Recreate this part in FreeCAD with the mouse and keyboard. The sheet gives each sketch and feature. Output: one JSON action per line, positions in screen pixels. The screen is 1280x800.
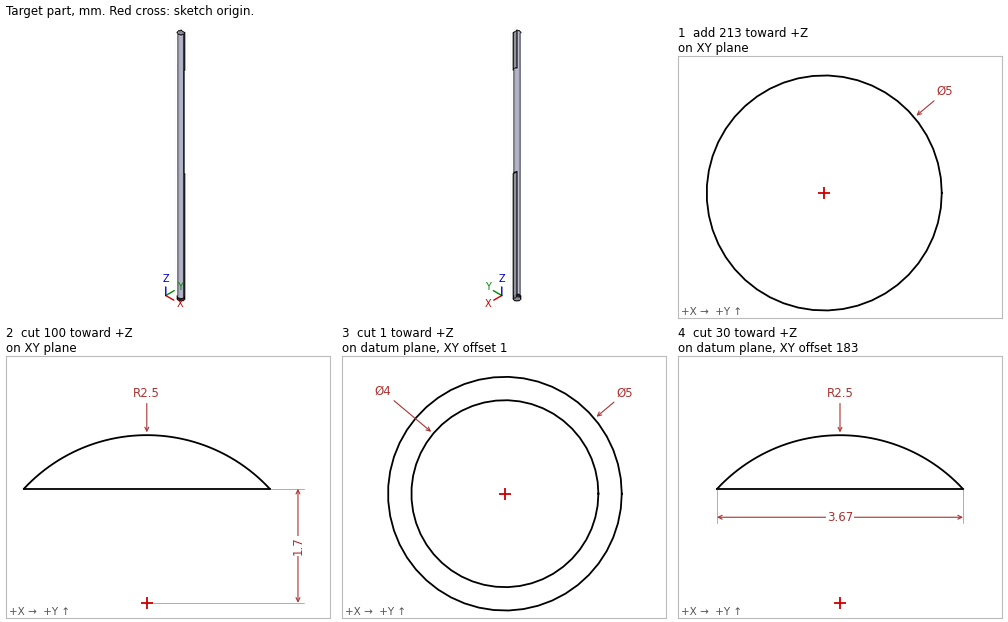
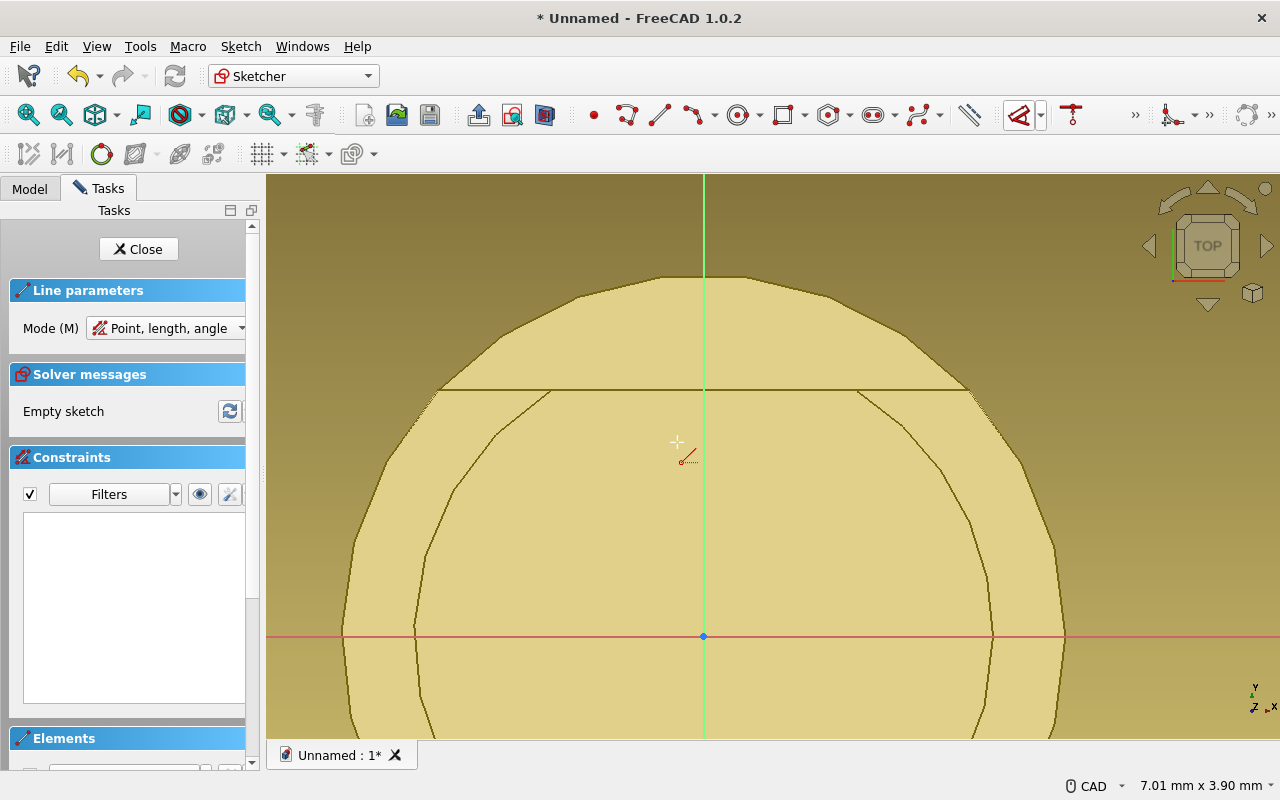
{"action": "left_click", "coordinate": [438, 391]}
{"action": "left_click", "coordinate": [969, 391]}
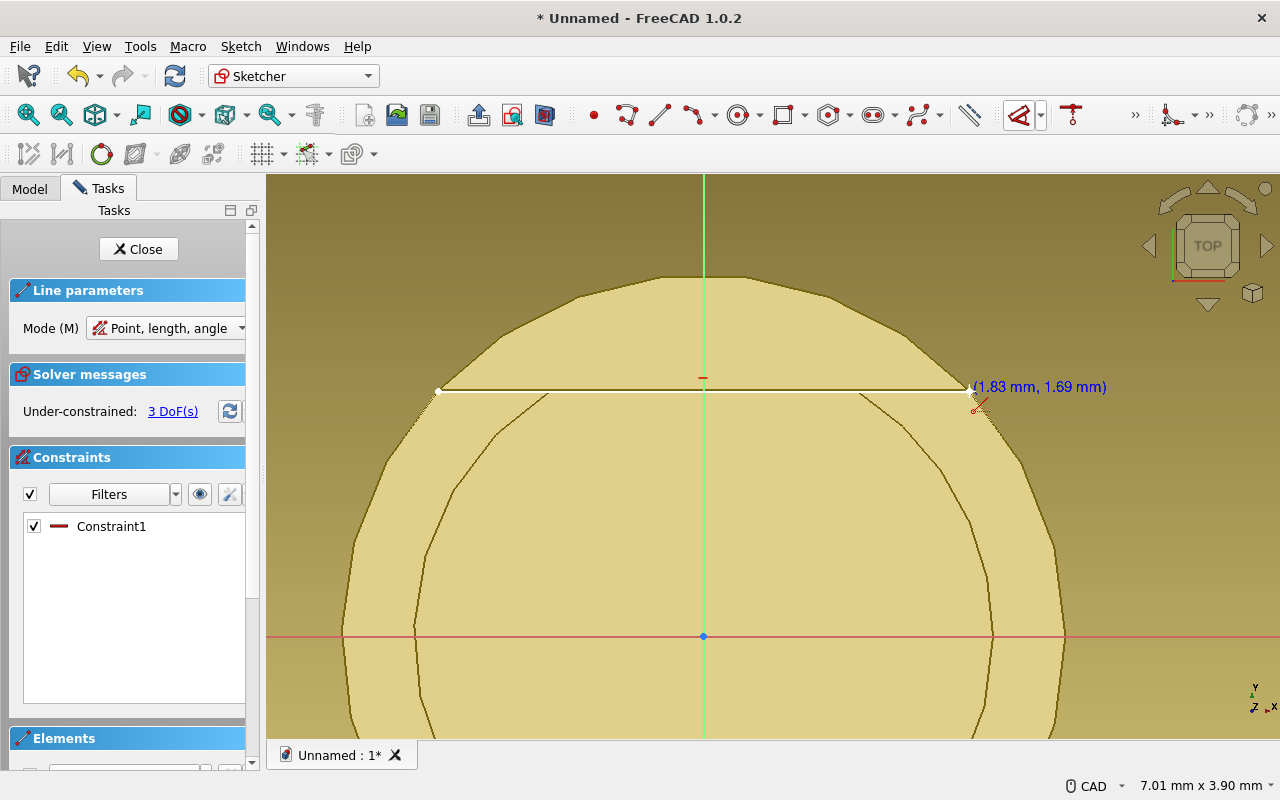
{"action": "key", "text": "g 3 a"}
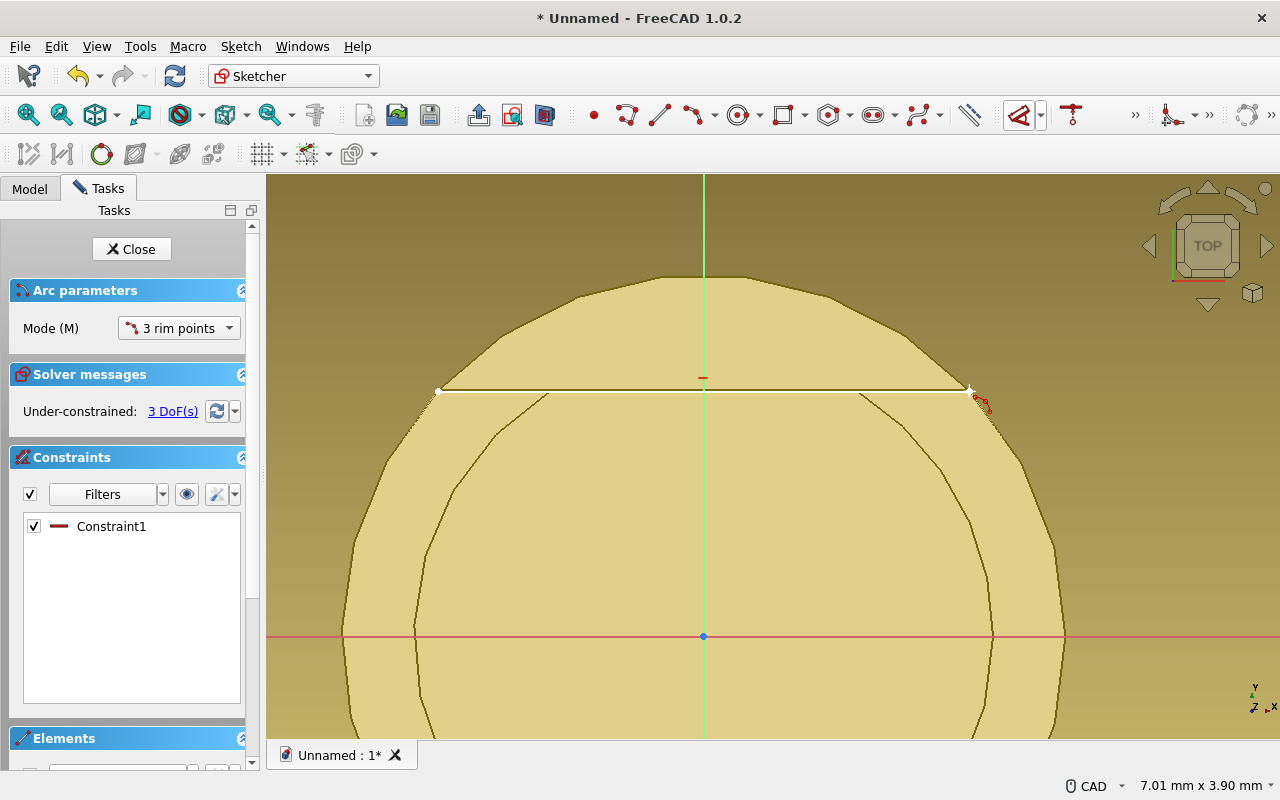
{"action": "left_click", "coordinate": [969, 392]}
{"action": "left_click", "coordinate": [438, 392]}
{"action": "left_click", "coordinate": [763, 280]}
{"action": "key", "text": "Escape"}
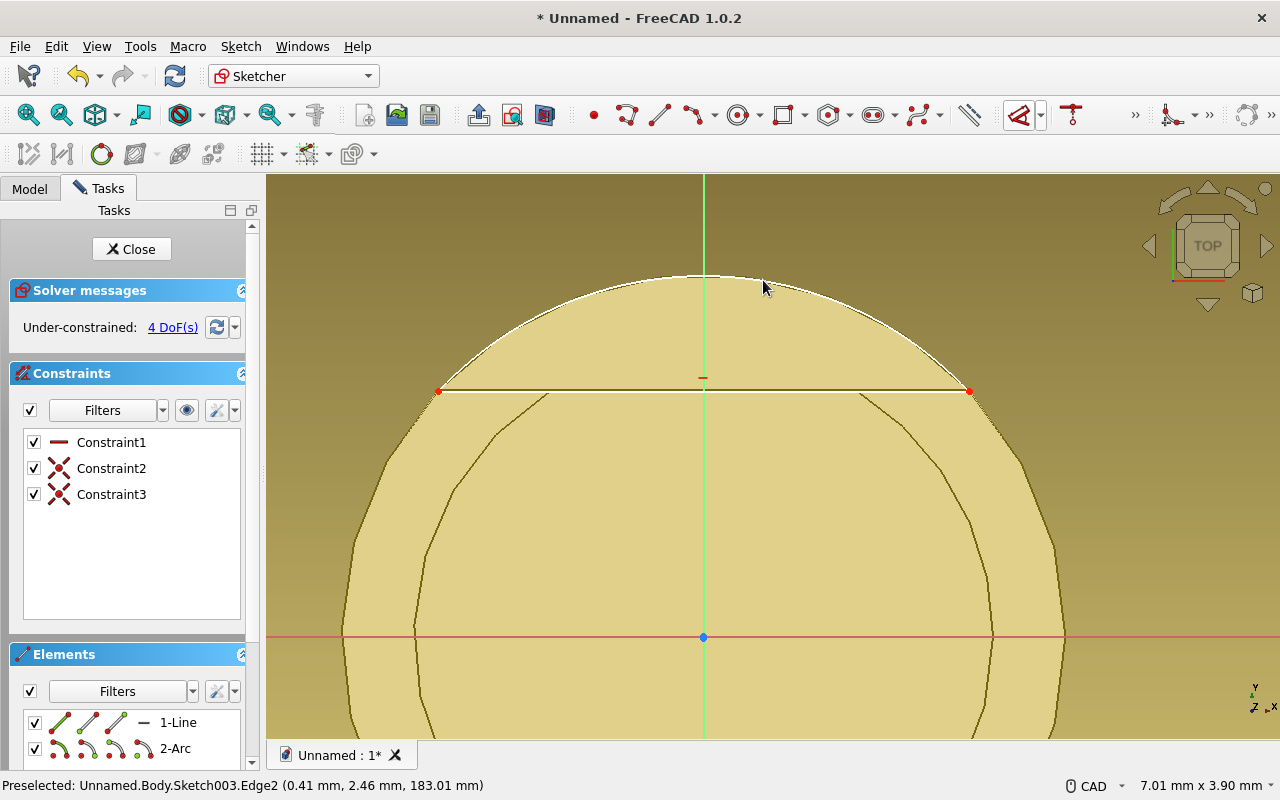
{"action": "left_click_drag", "start_coordinate": [694, 627], "coordinate": [714, 648]}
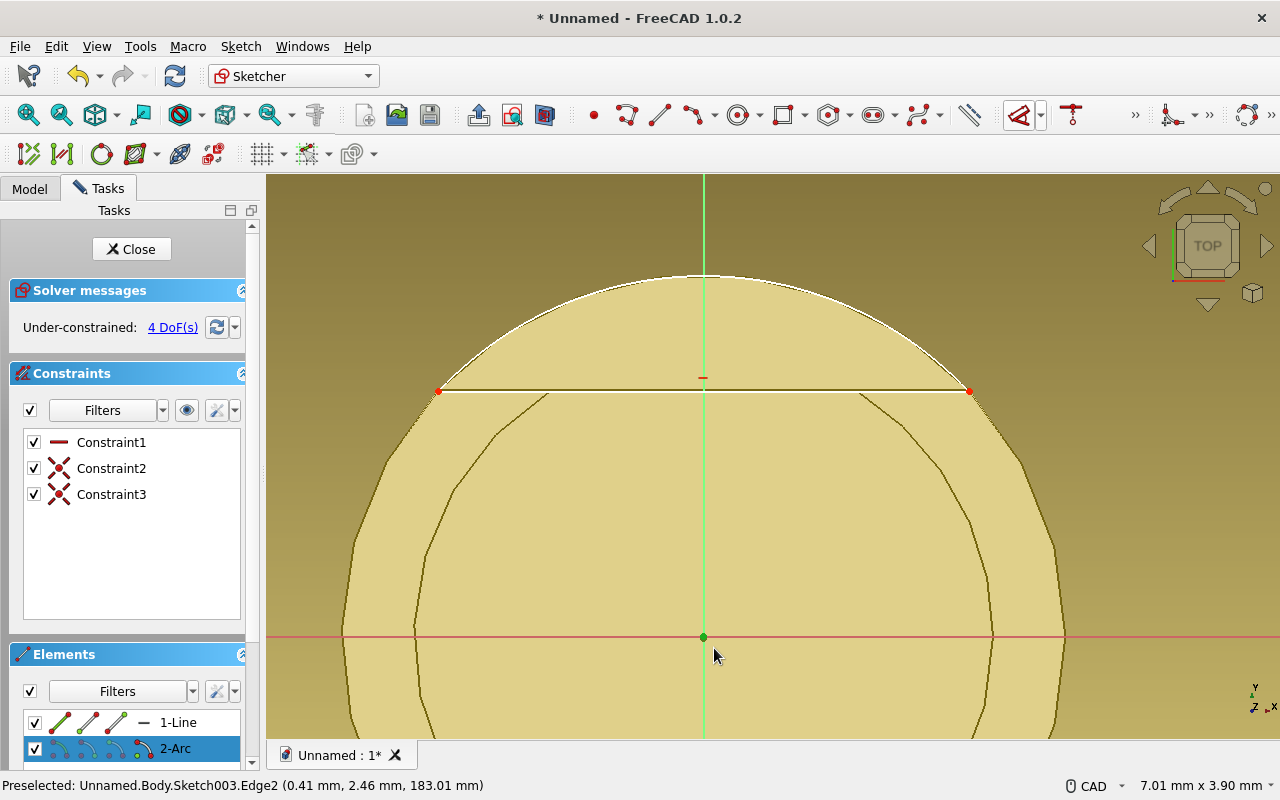
{"action": "key", "text": "c"}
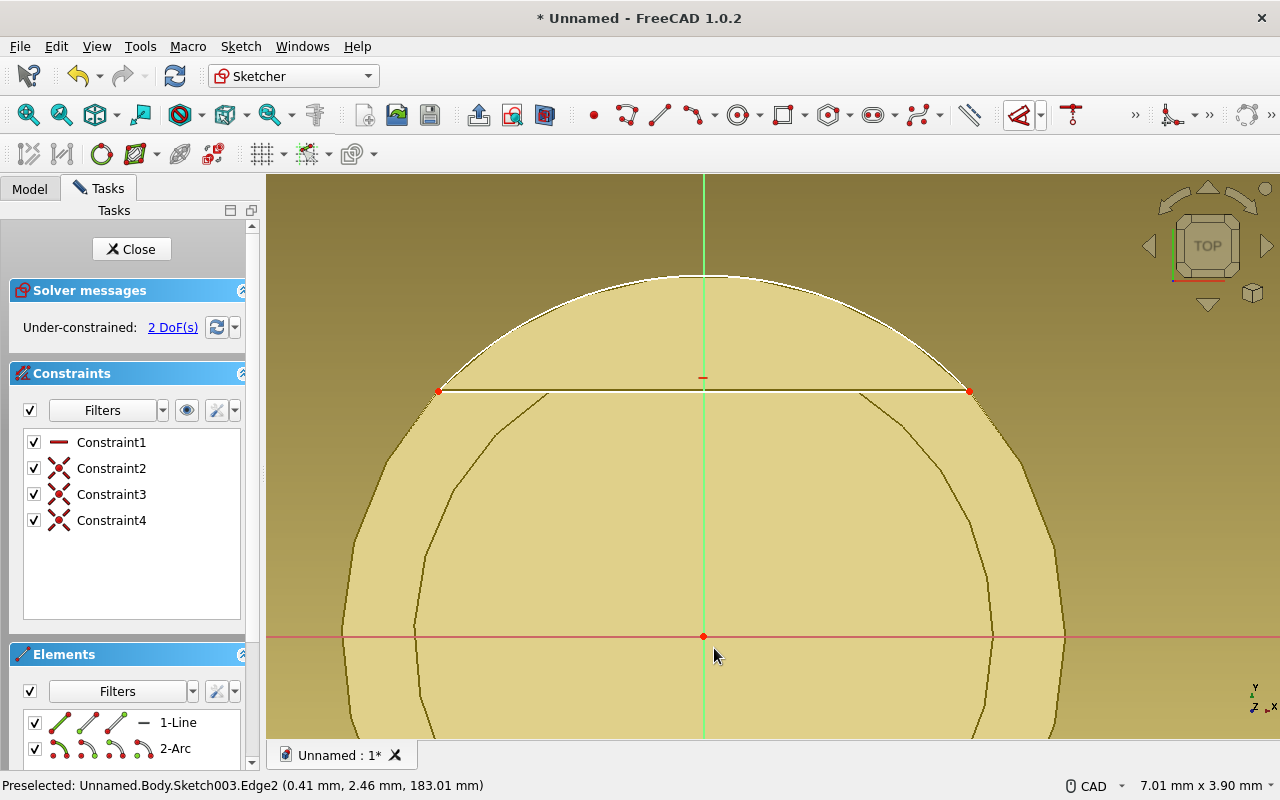
{"action": "left_click", "coordinate": [821, 295]}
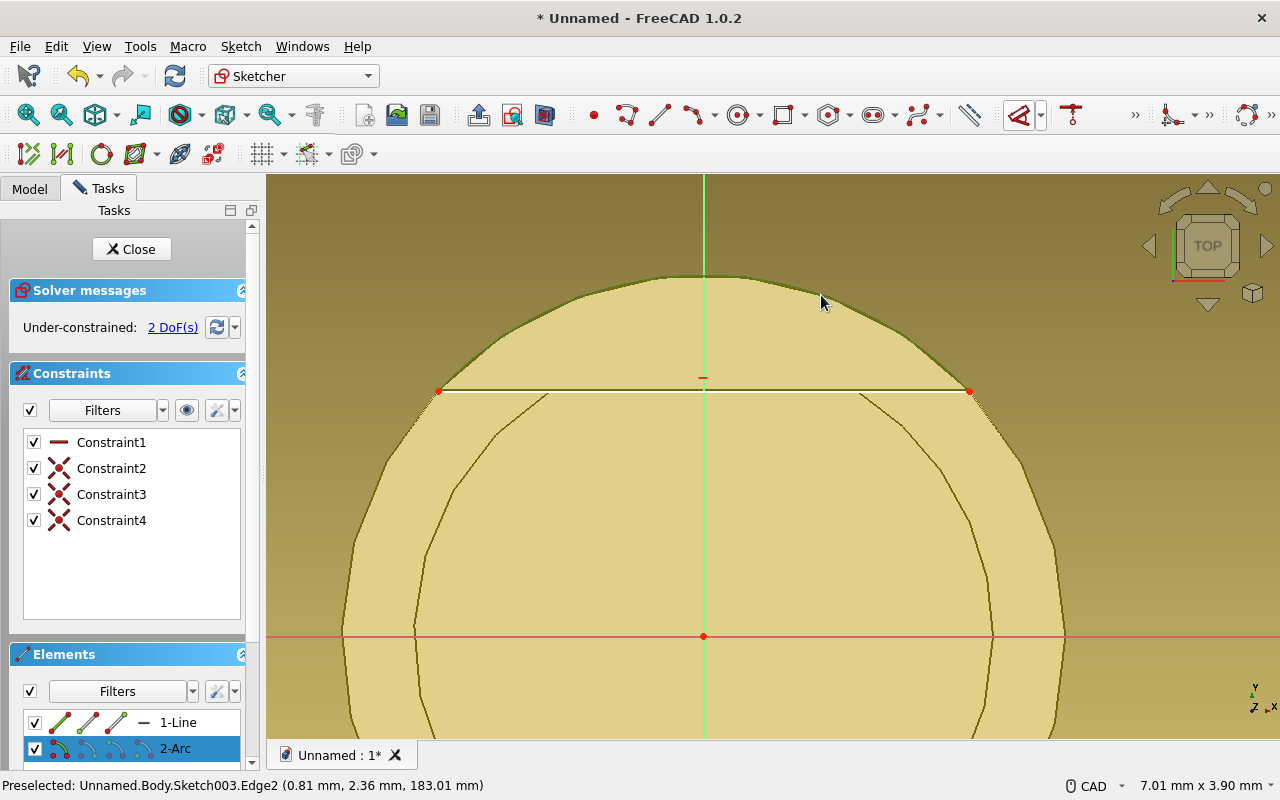
{"action": "key", "text": "k r"}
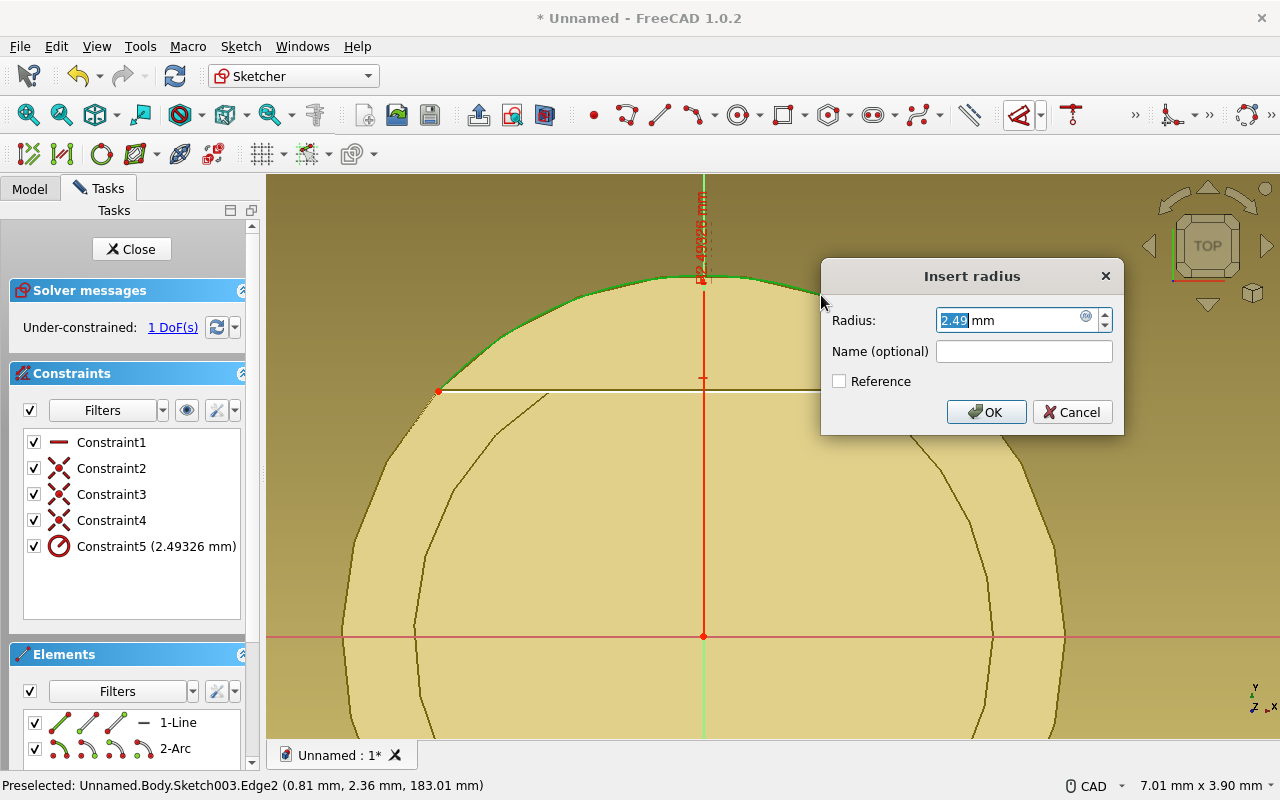
{"action": "type", "text": "2.5"}
{"action": "key", "text": "Return"}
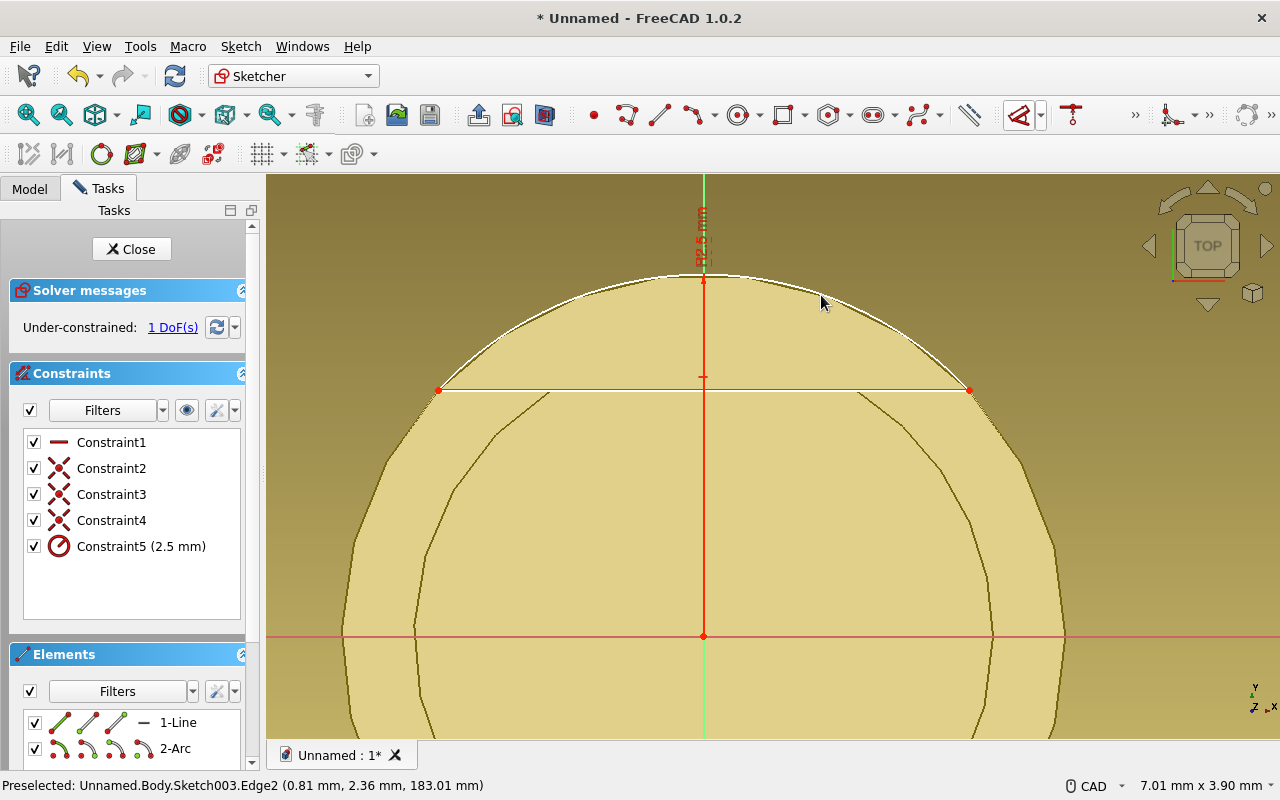
{"action": "left_click", "coordinate": [597, 391]}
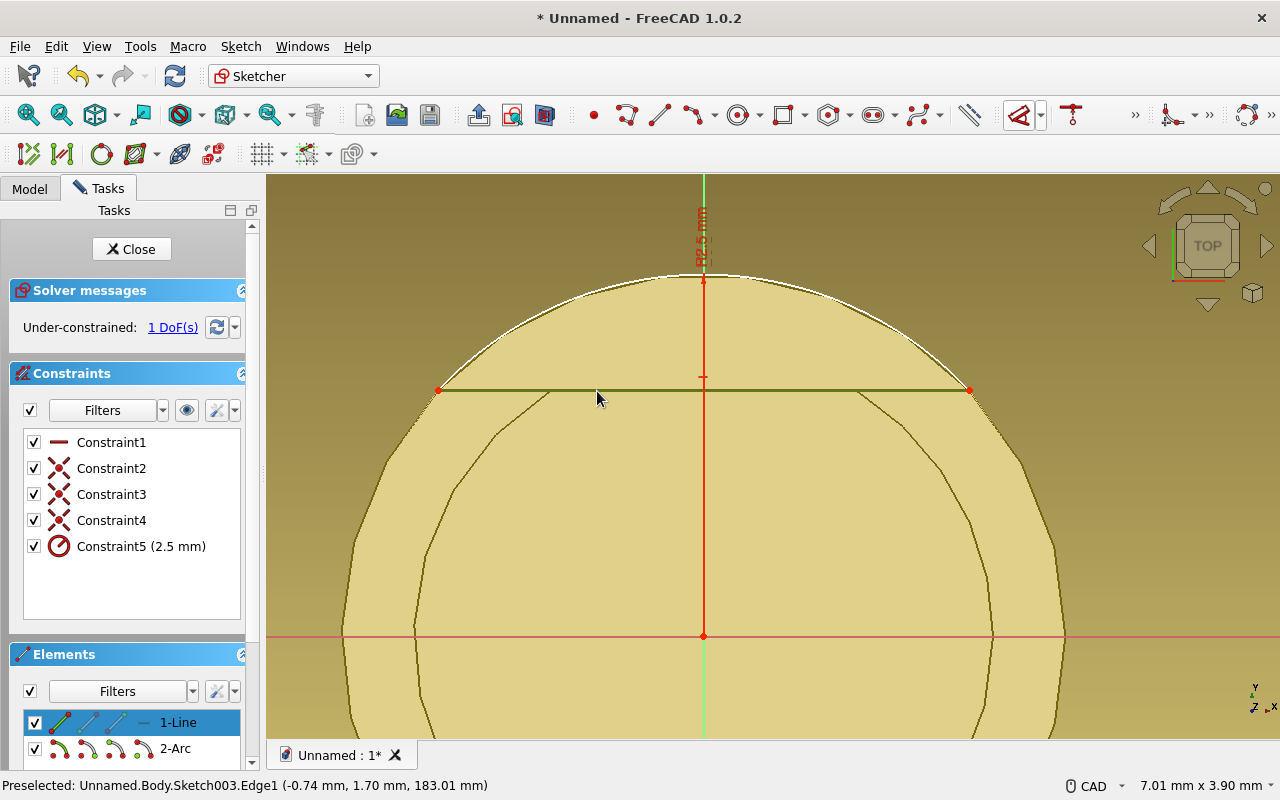
{"action": "key", "text": "l"}